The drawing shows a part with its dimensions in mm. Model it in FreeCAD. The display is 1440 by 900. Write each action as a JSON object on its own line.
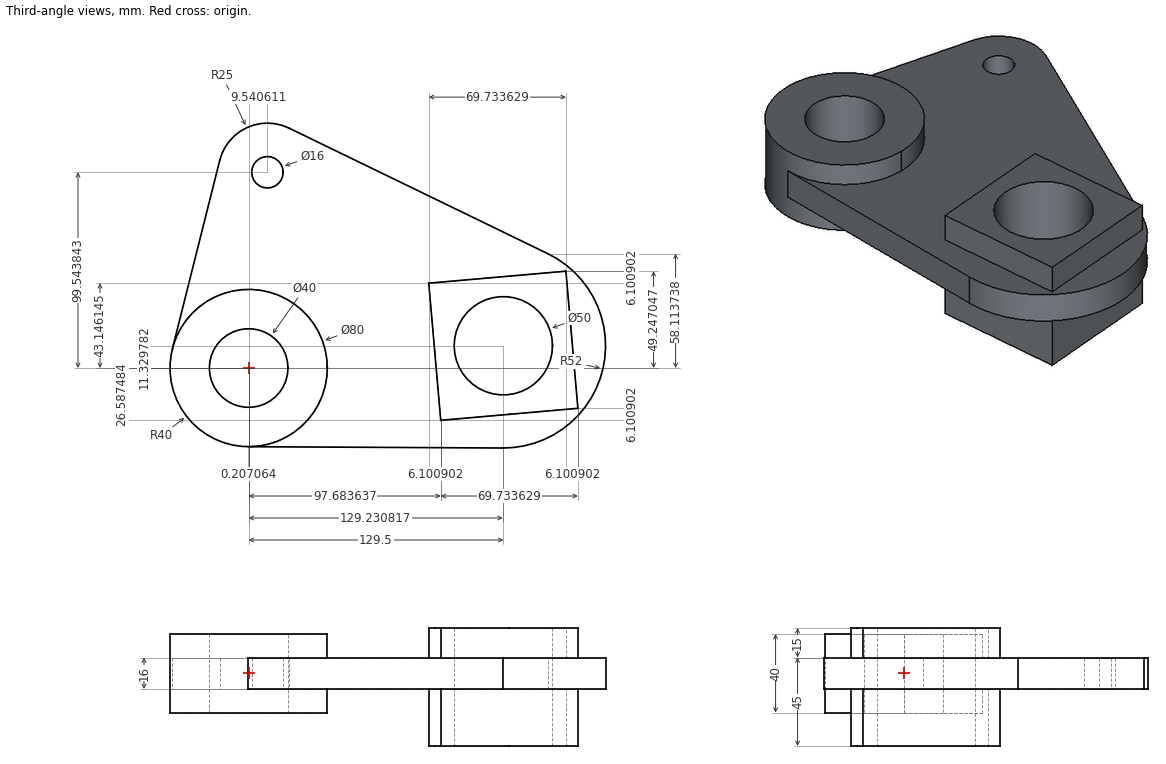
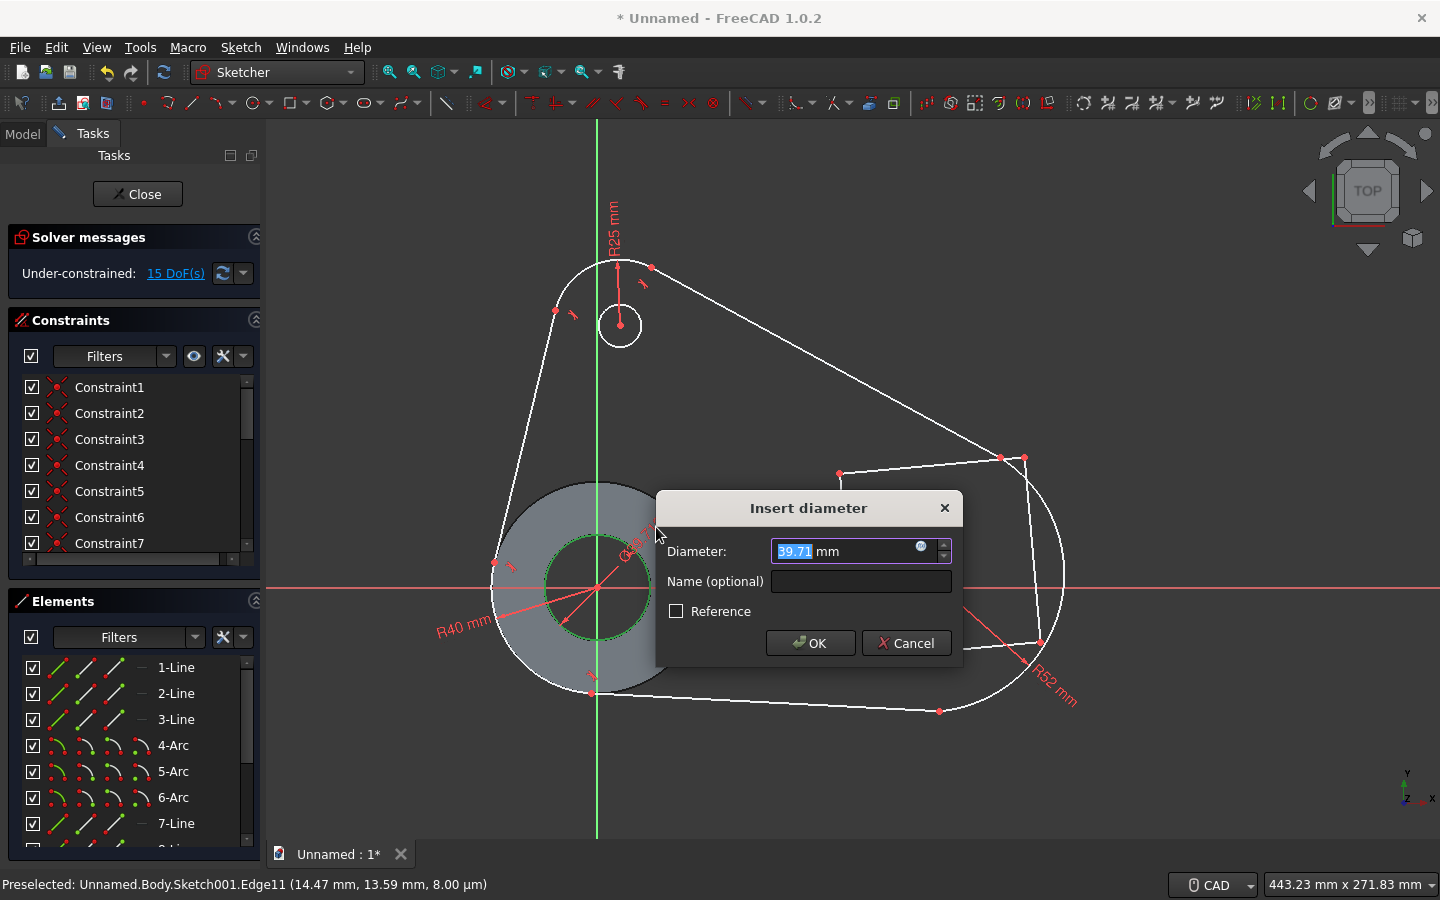
{"action": "type", "text": "40"}
{"action": "key", "text": "Return"}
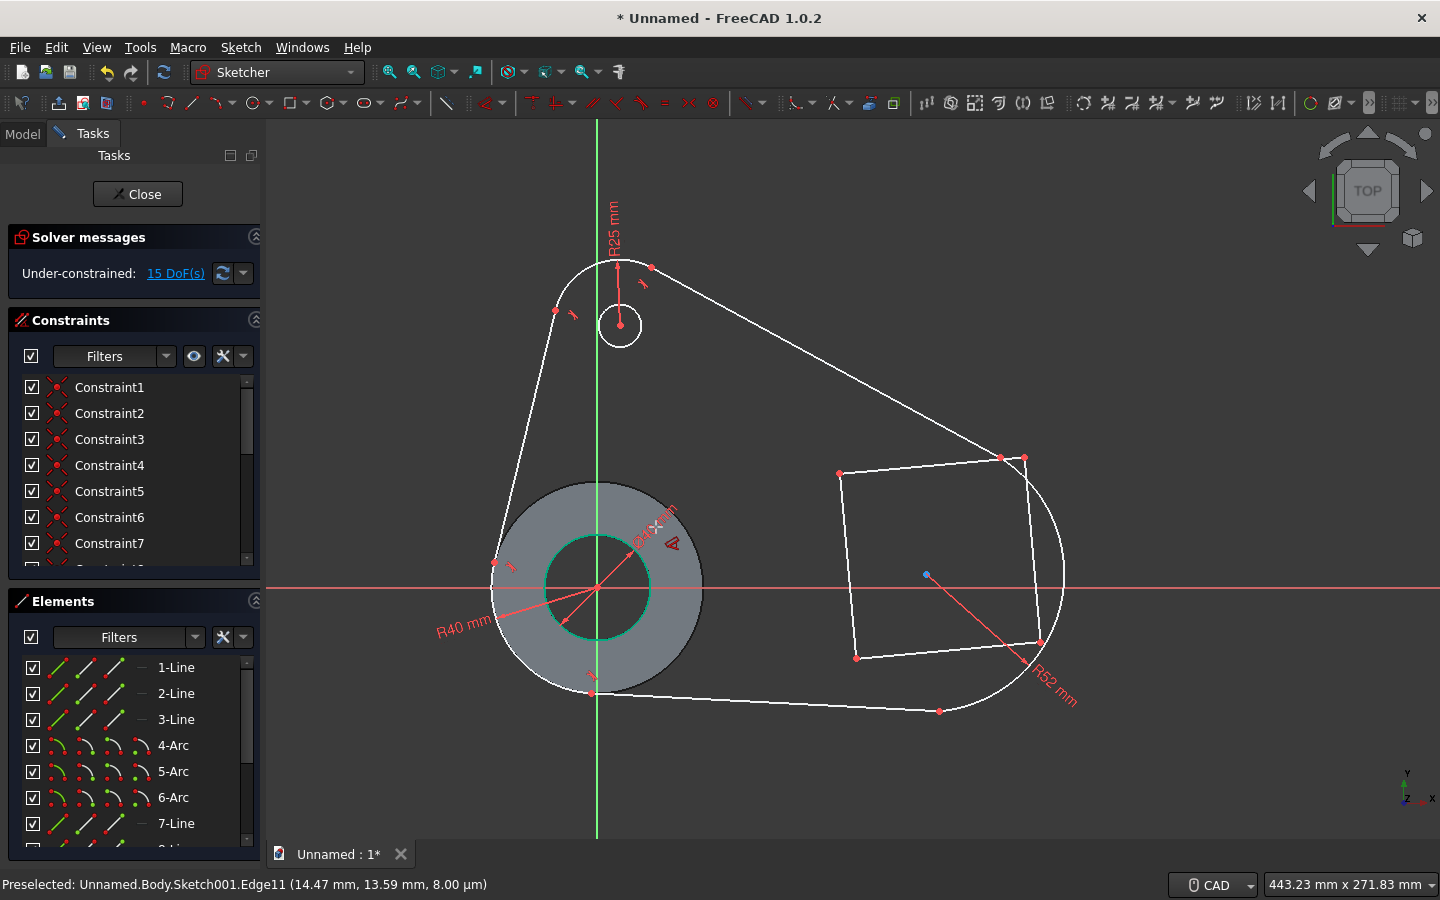
{"action": "left_click", "coordinate": [635, 311]}
{"action": "left_click", "coordinate": [658, 288]}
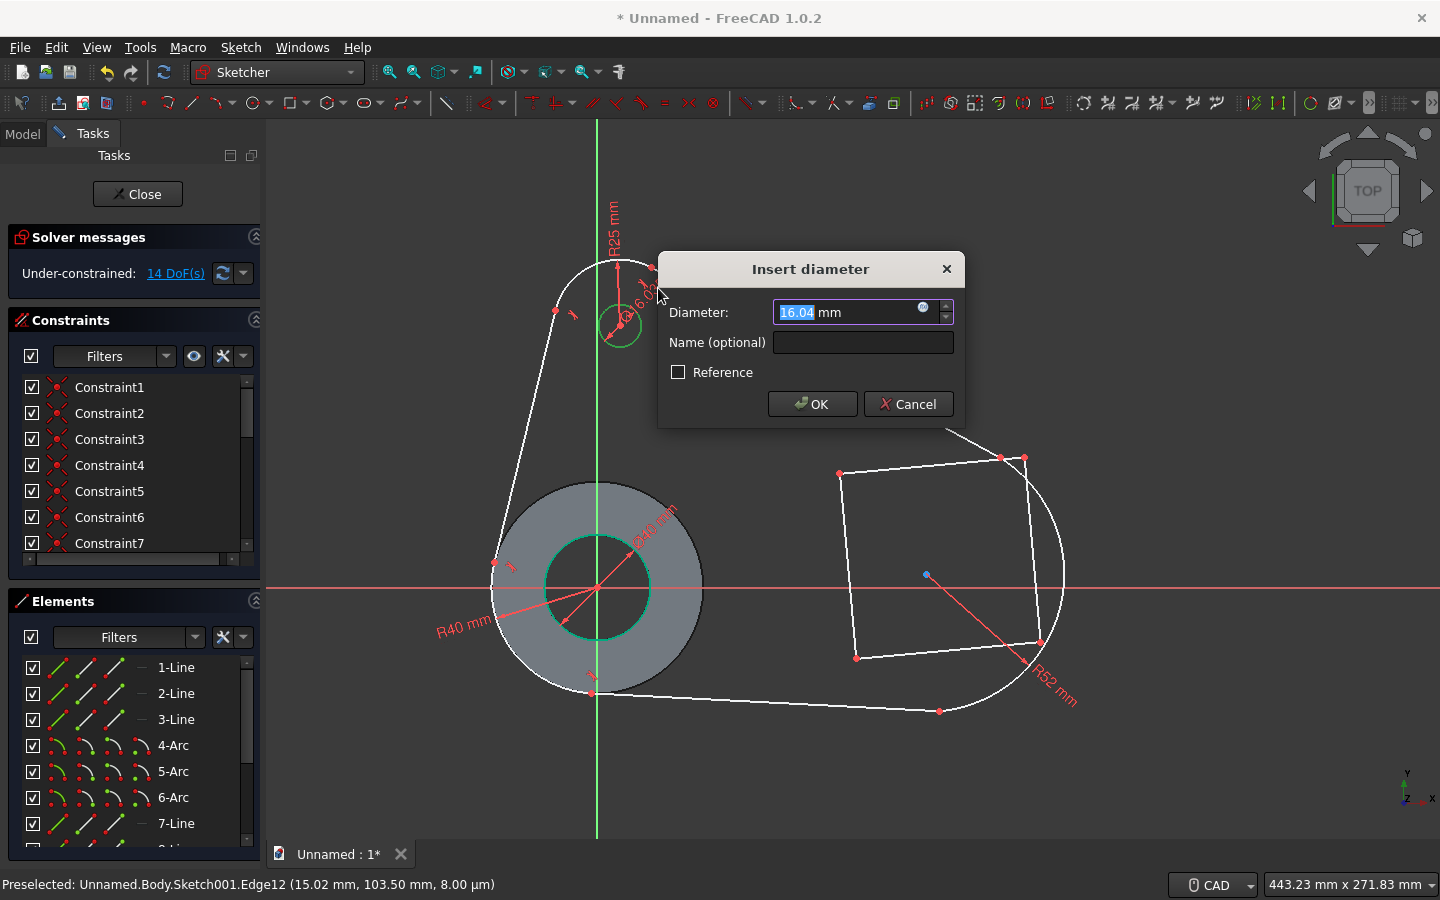
{"action": "type", "text": "16"}
{"action": "key", "text": "Return"}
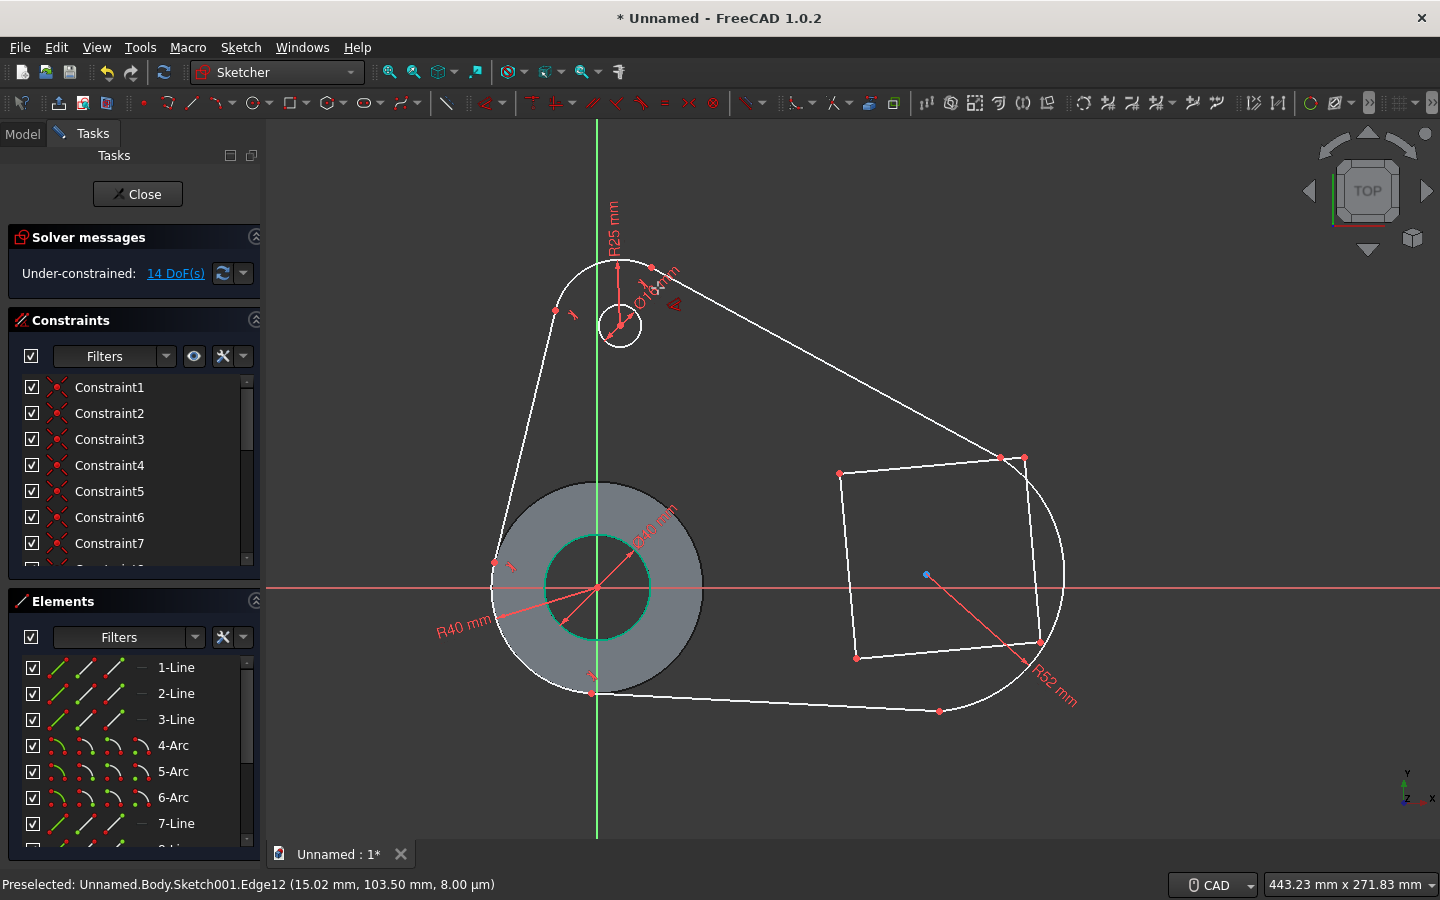
{"action": "left_click", "coordinate": [926, 574]}
{"action": "left_click", "coordinate": [762, 622]}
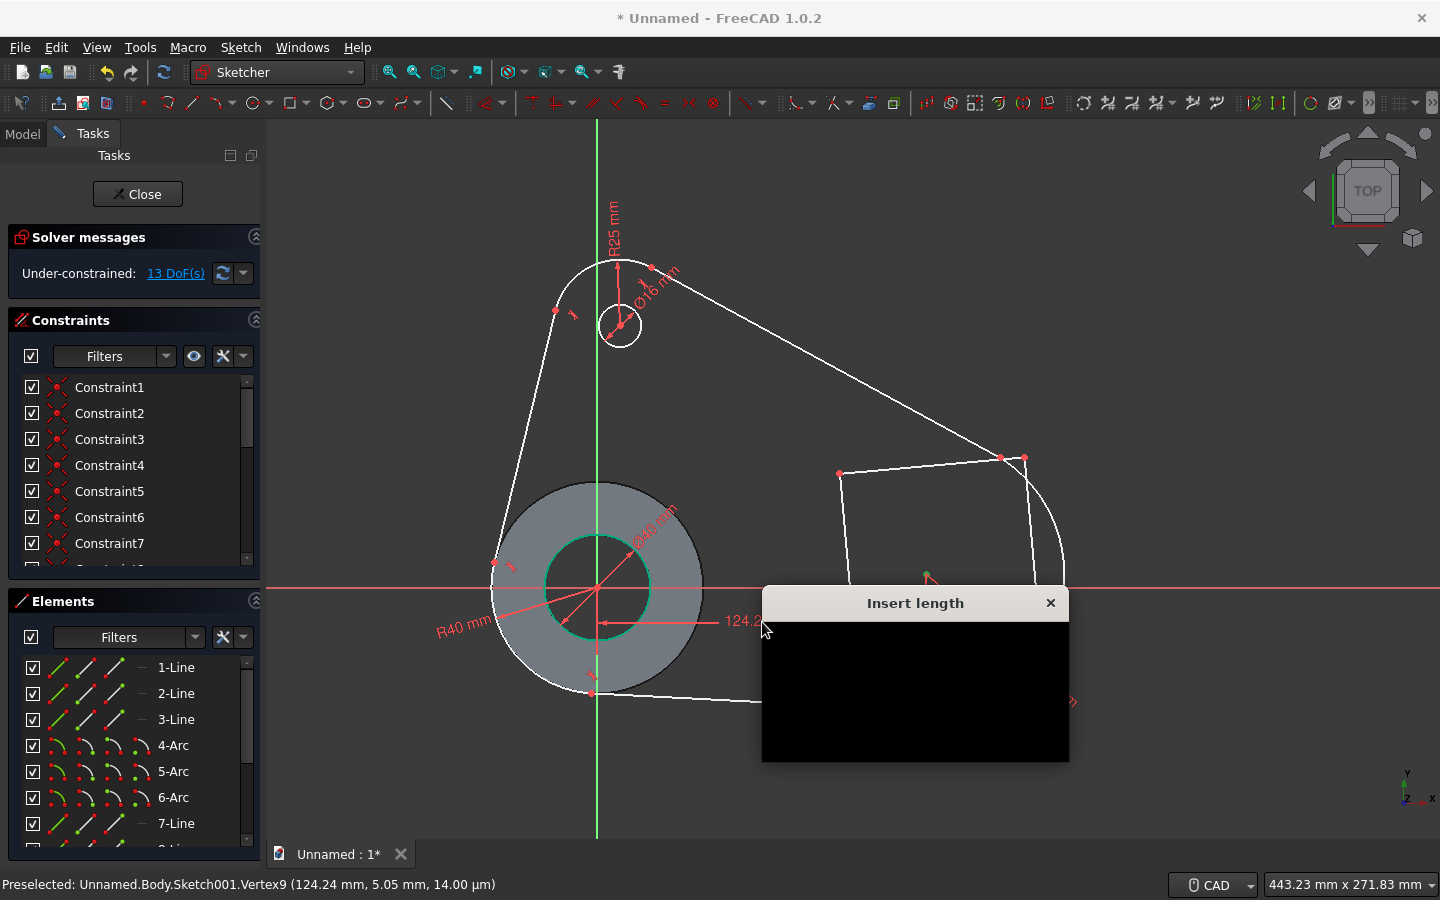
{"action": "type", "text": "129.5"}
{"action": "key", "text": "Return"}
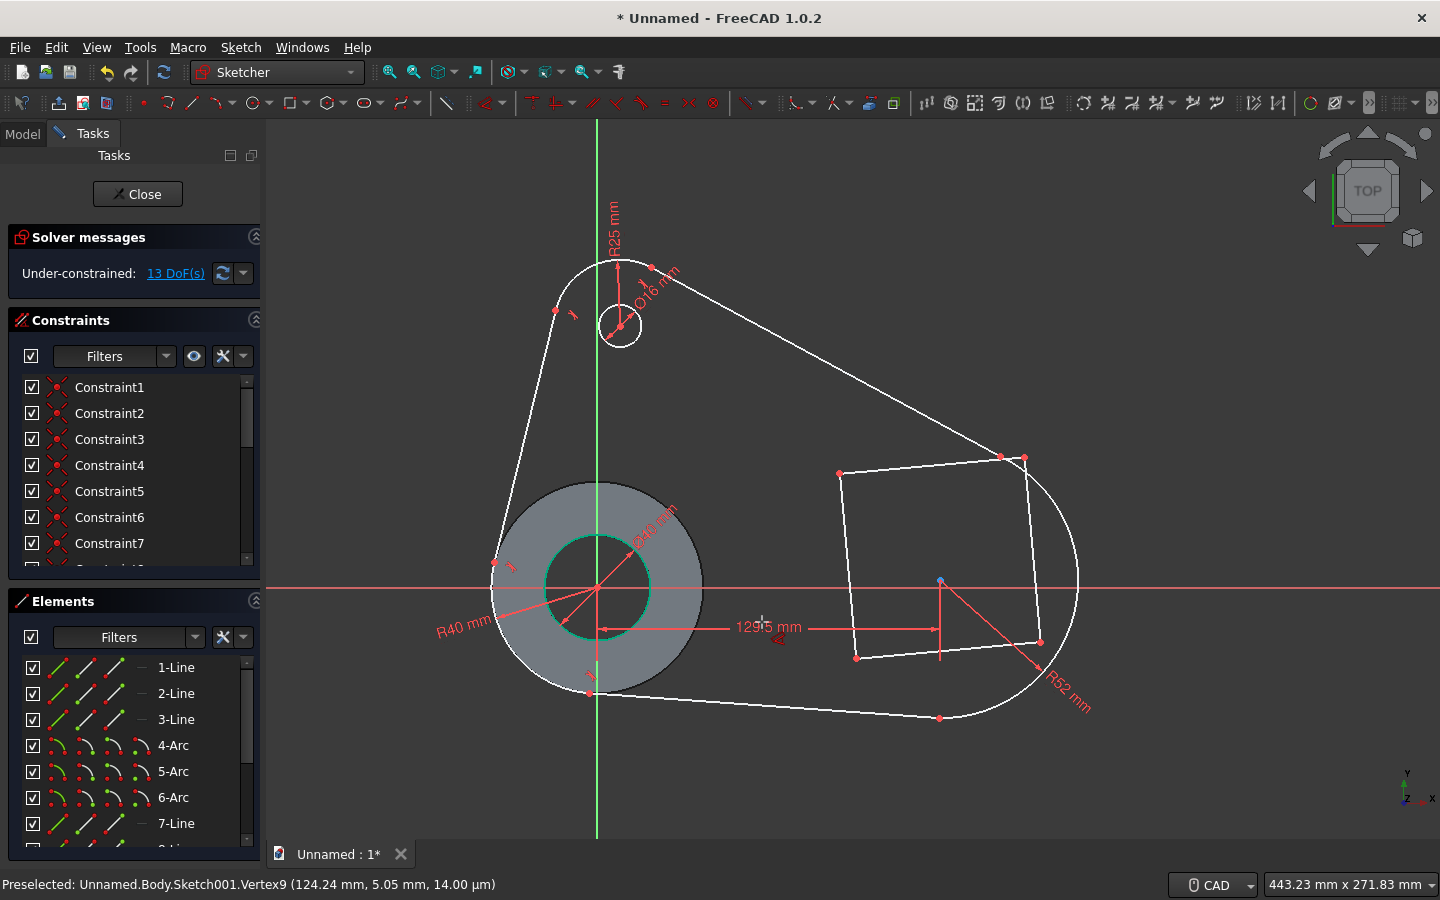
{"action": "scroll", "coordinate": [620, 326], "scroll_direction": "up", "scroll_amount": 3}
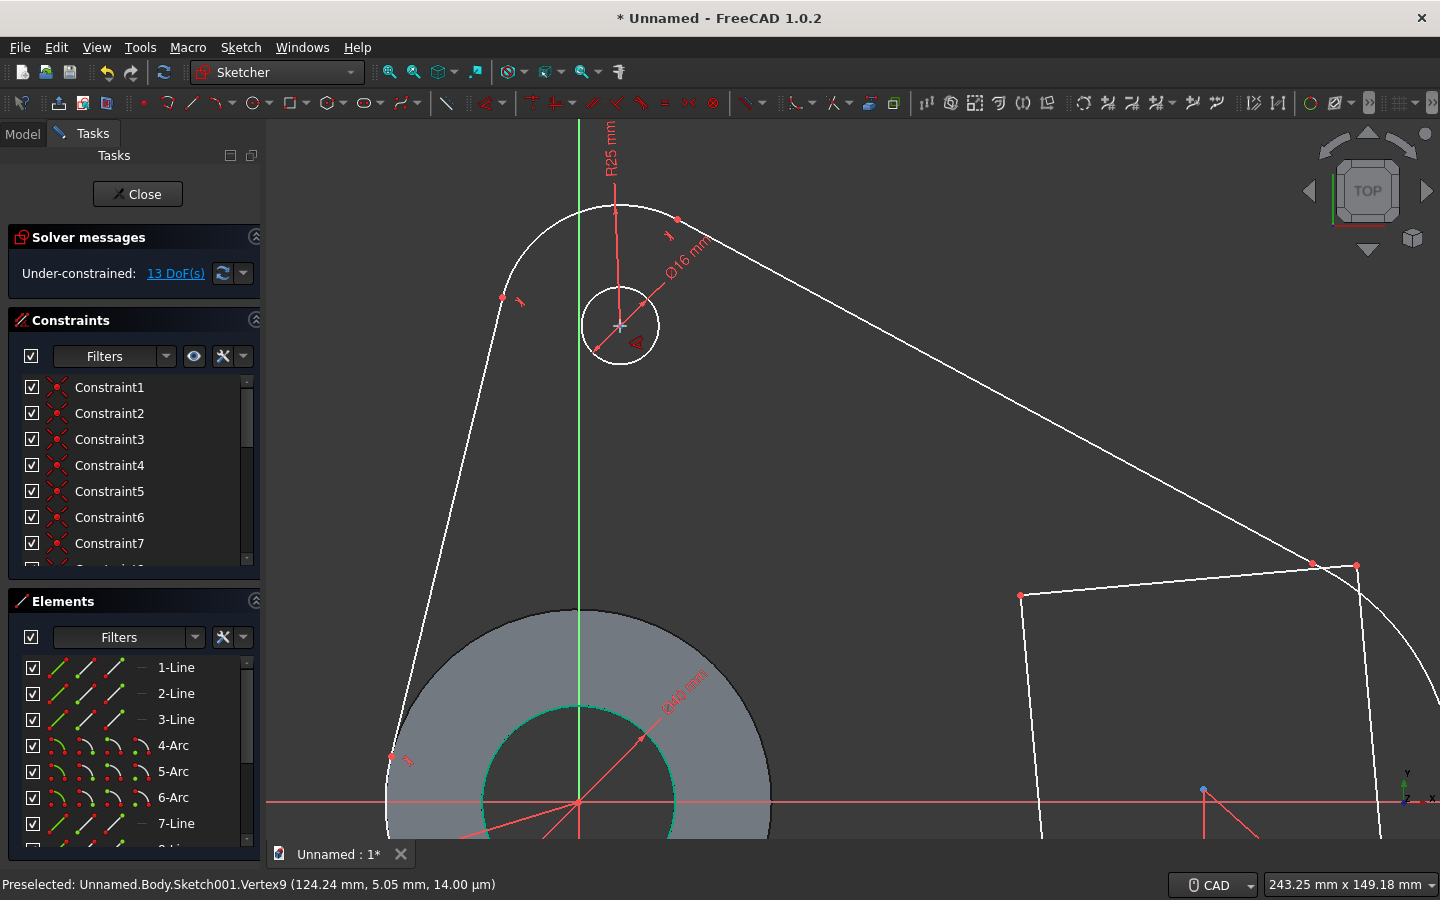
{"action": "left_click", "coordinate": [620, 326]}
{"action": "left_click", "coordinate": [599, 268]}